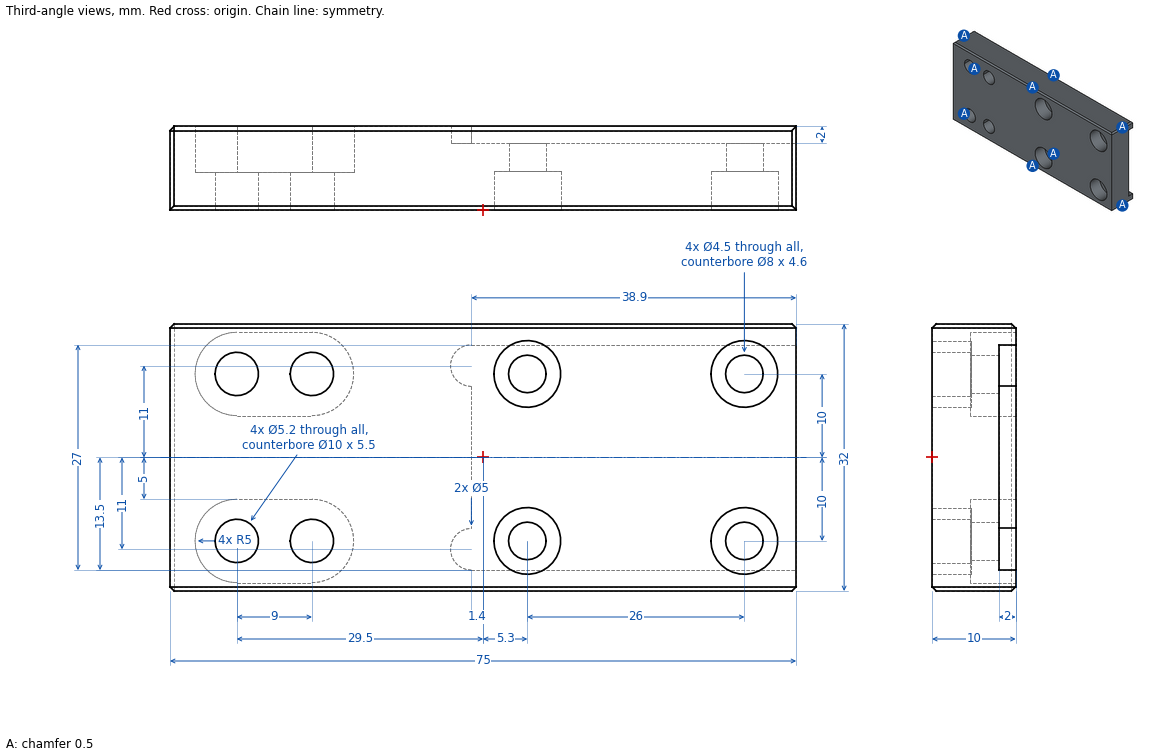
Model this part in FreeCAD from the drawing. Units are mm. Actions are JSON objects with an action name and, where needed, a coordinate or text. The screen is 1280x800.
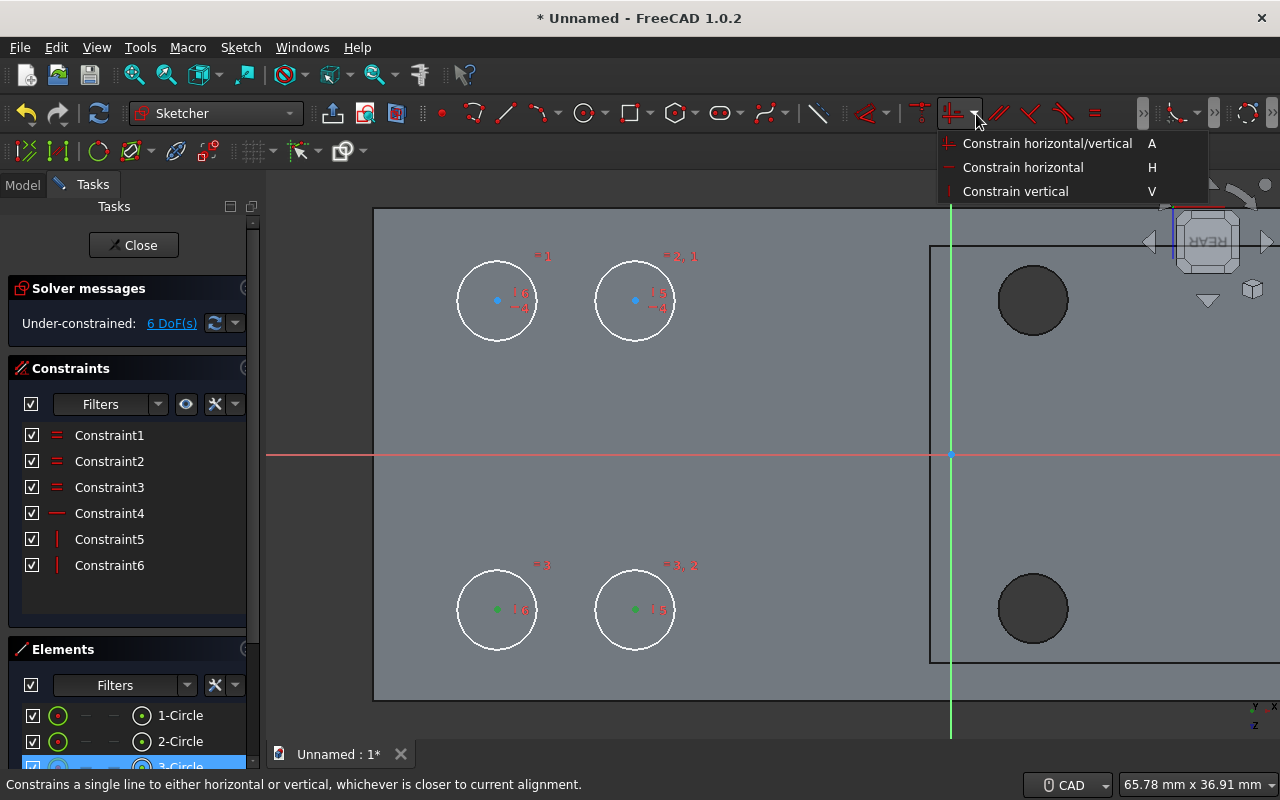
{"action": "left_click", "coordinate": [1073, 167]}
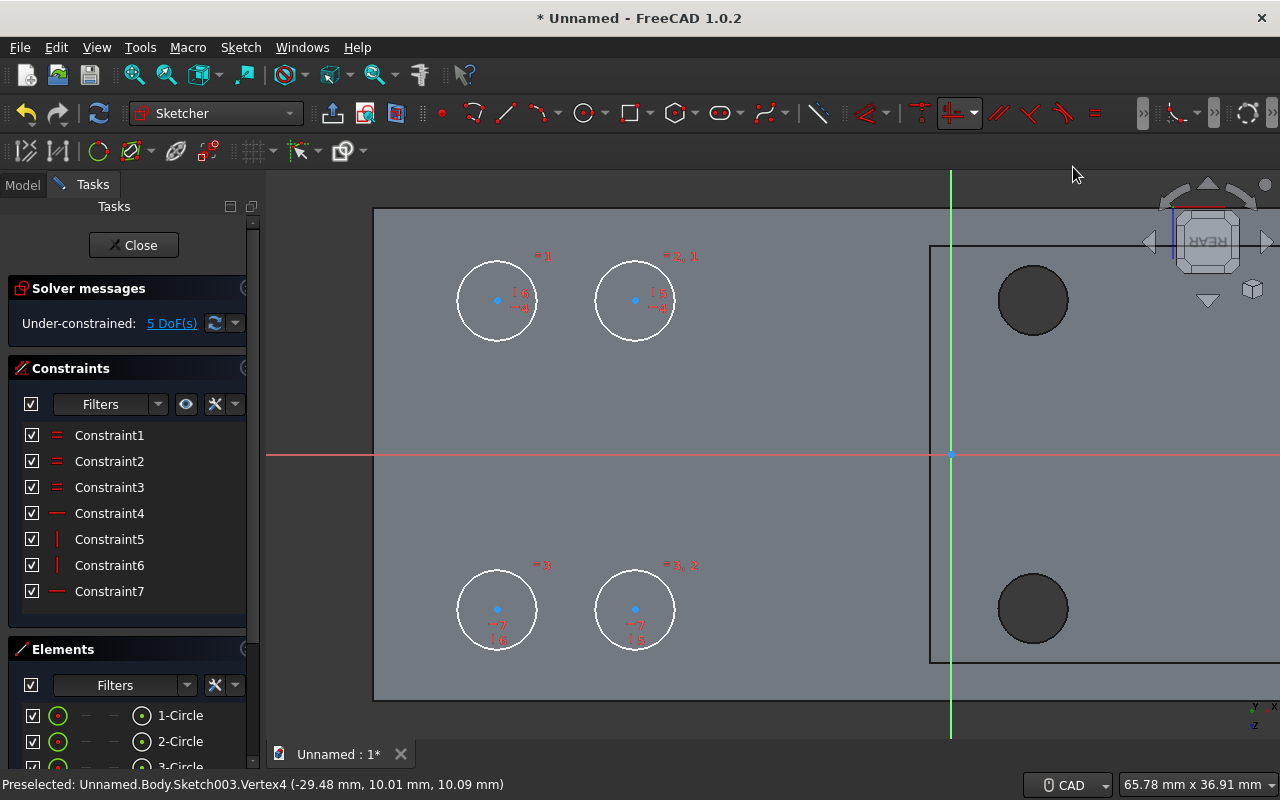
{"action": "left_click", "coordinate": [866, 114]}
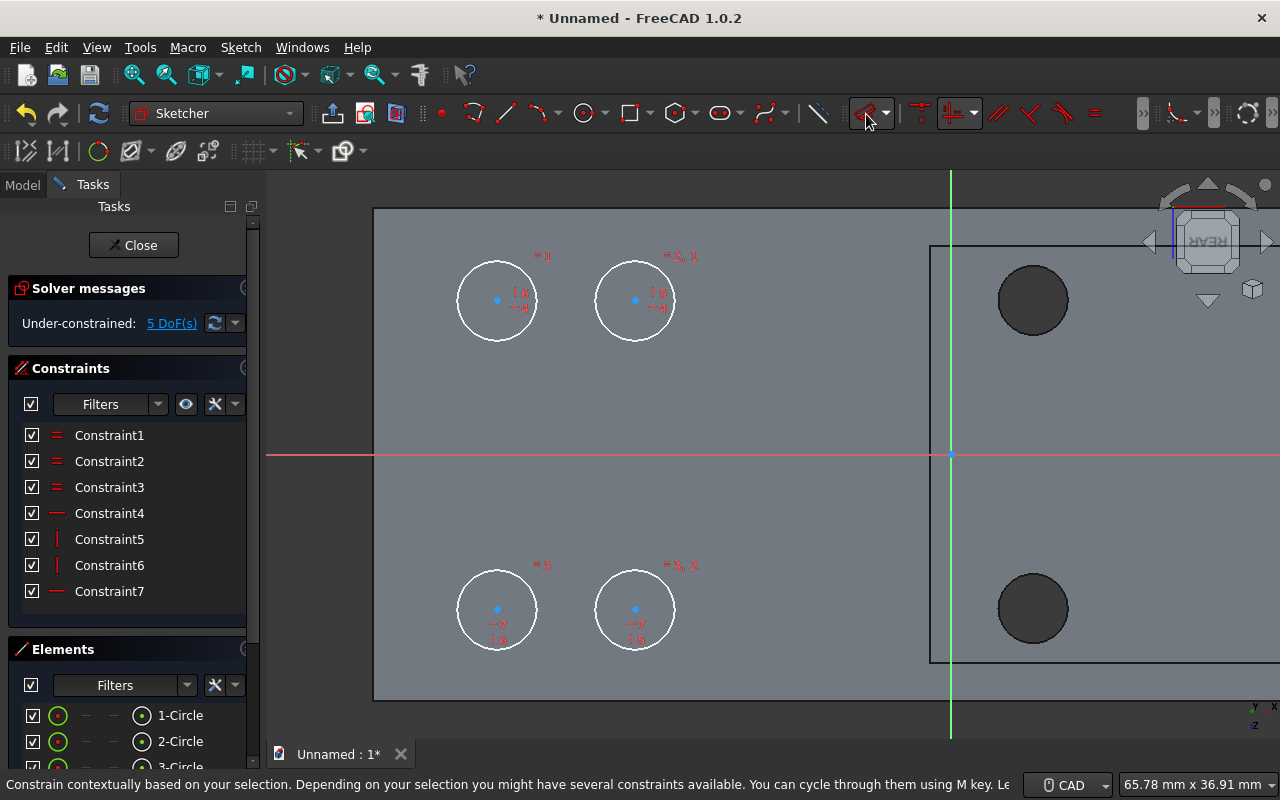
{"action": "left_click", "coordinate": [525, 273]}
{"action": "left_click", "coordinate": [548, 250]}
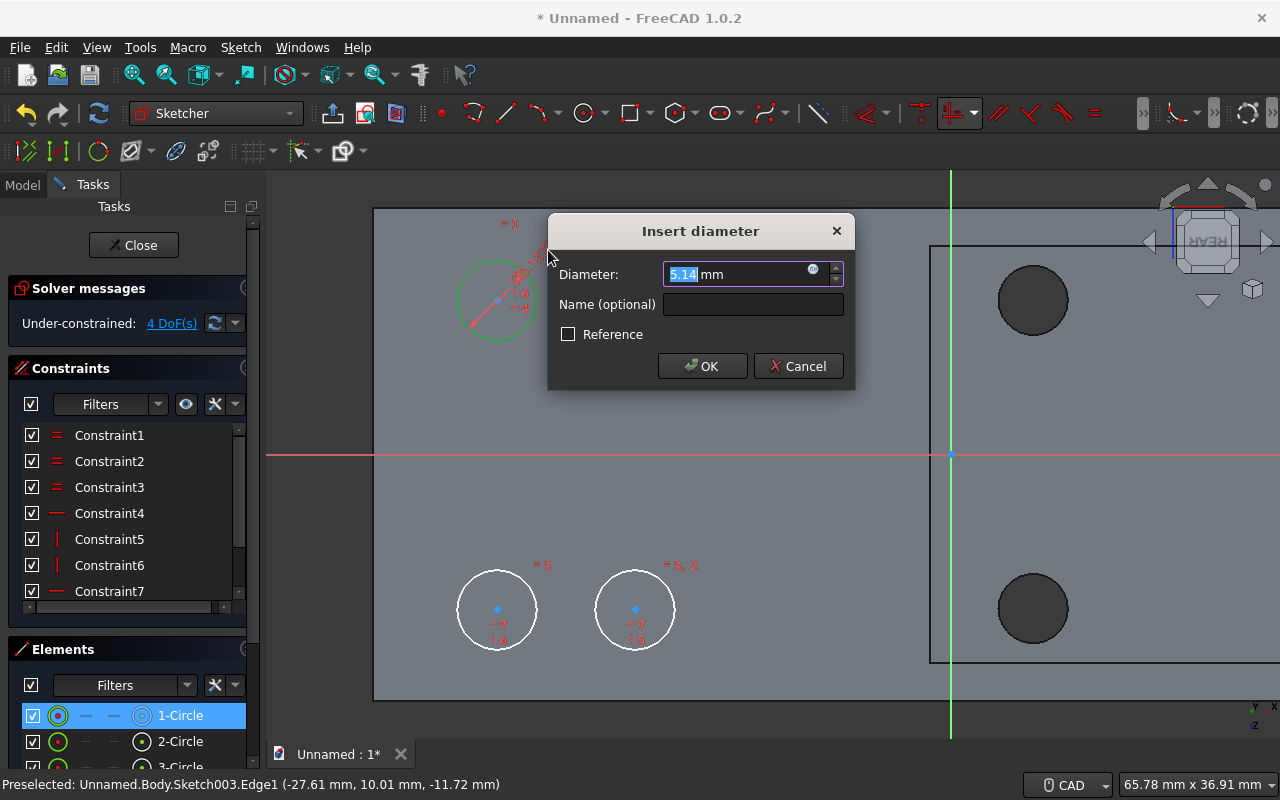
{"action": "type", "text": "5.2"}
{"action": "key", "text": "Return"}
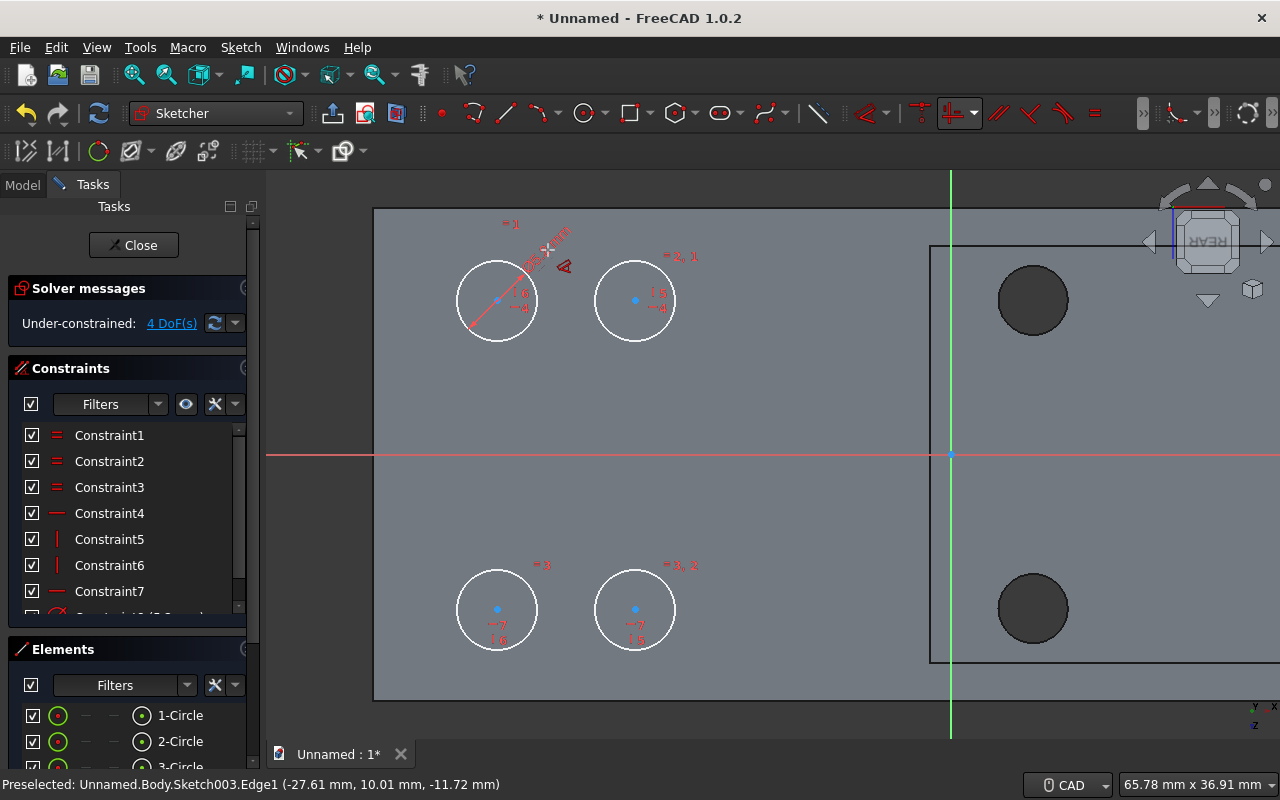
{"action": "left_click", "coordinate": [497, 301]}
{"action": "left_click", "coordinate": [985, 378]}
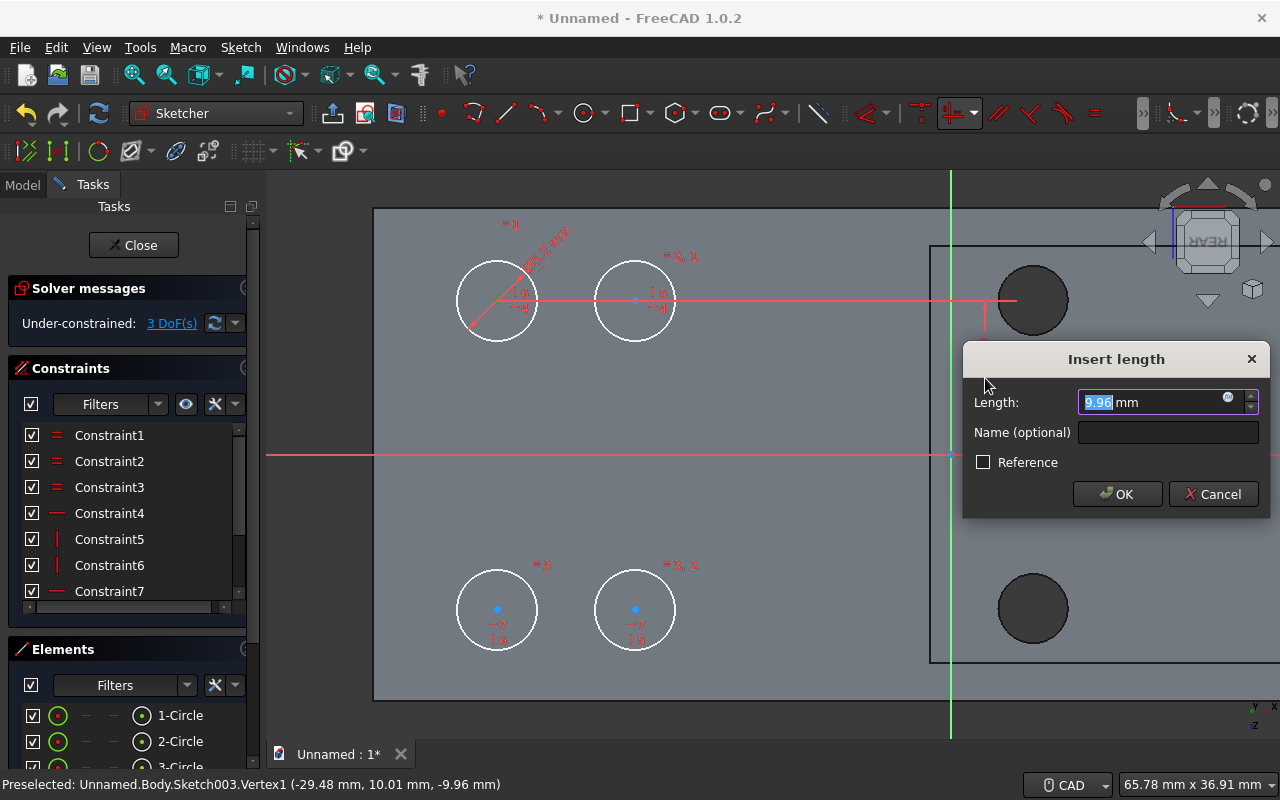
{"action": "type", "text": "10"}
{"action": "key", "text": "Return"}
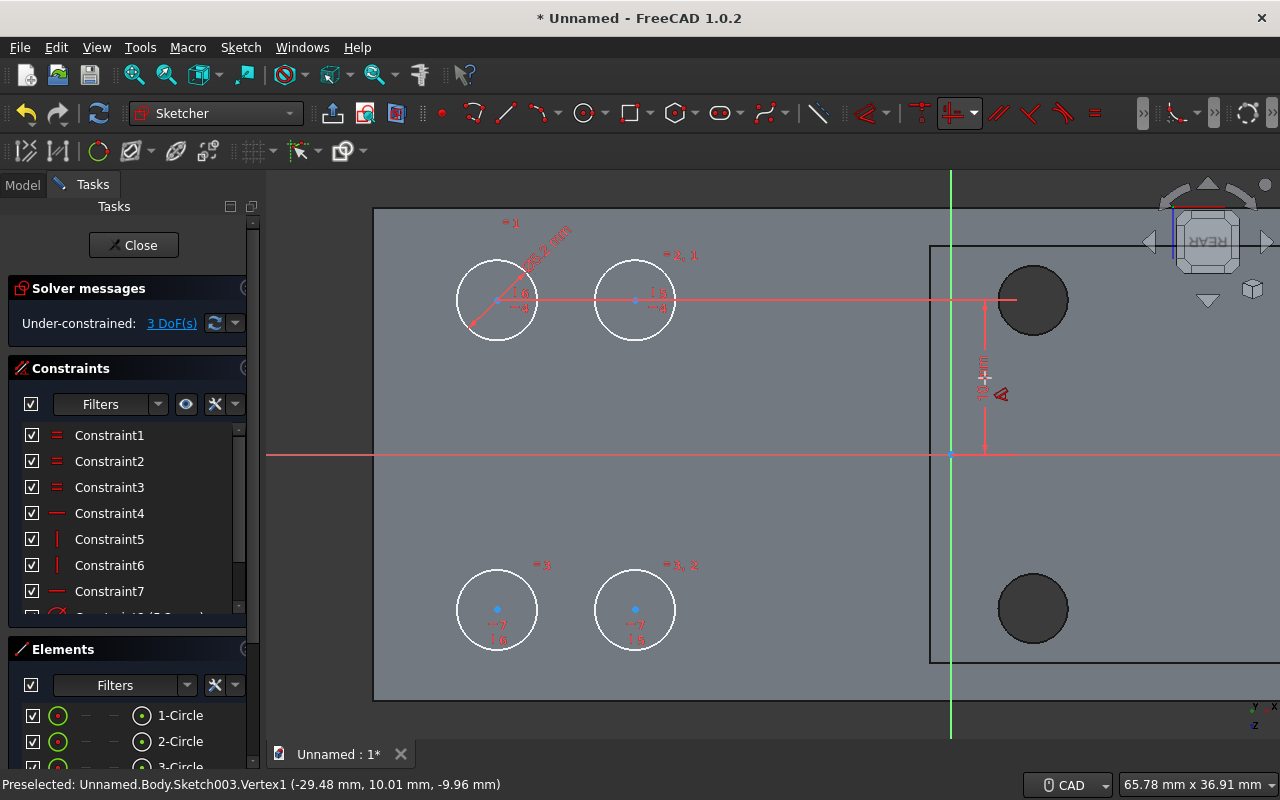
{"action": "left_click", "coordinate": [635, 610]}
{"action": "left_click", "coordinate": [985, 532]}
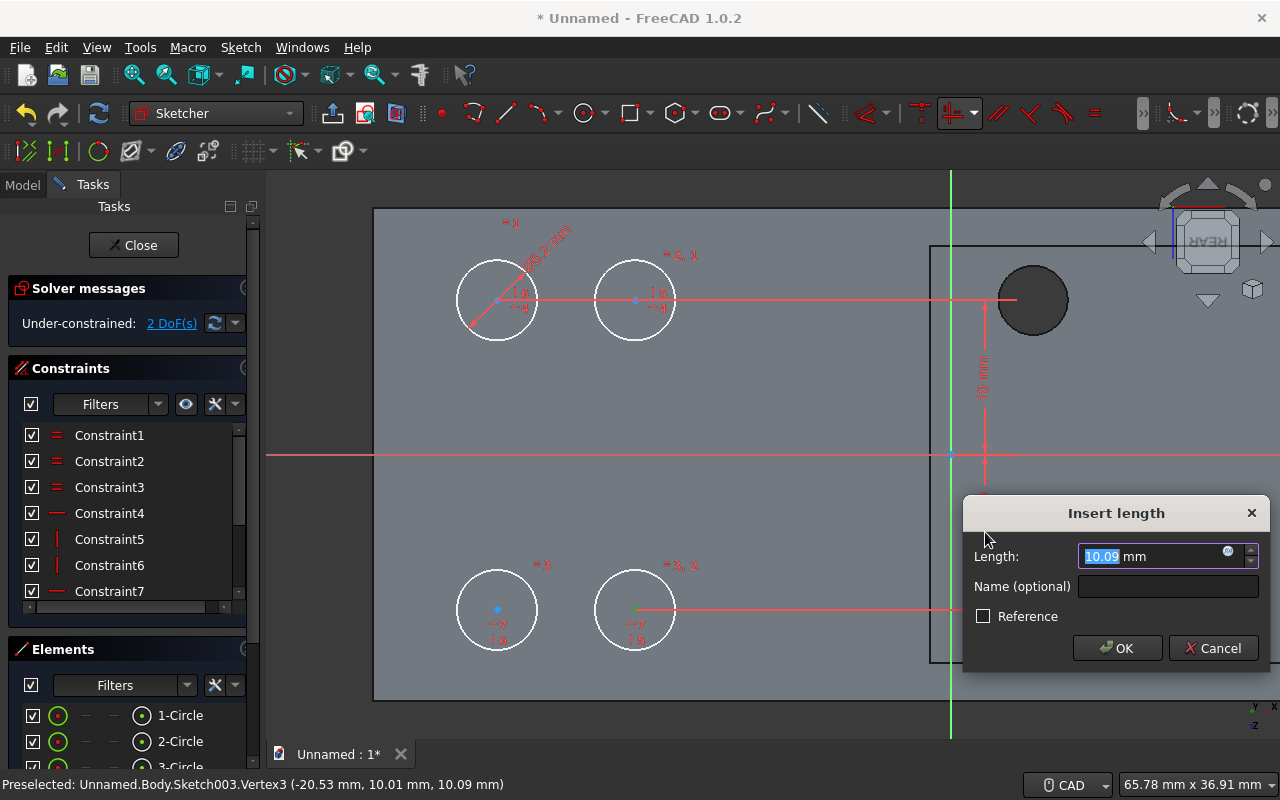
{"action": "type", "text": "10"}
{"action": "key", "text": "Return"}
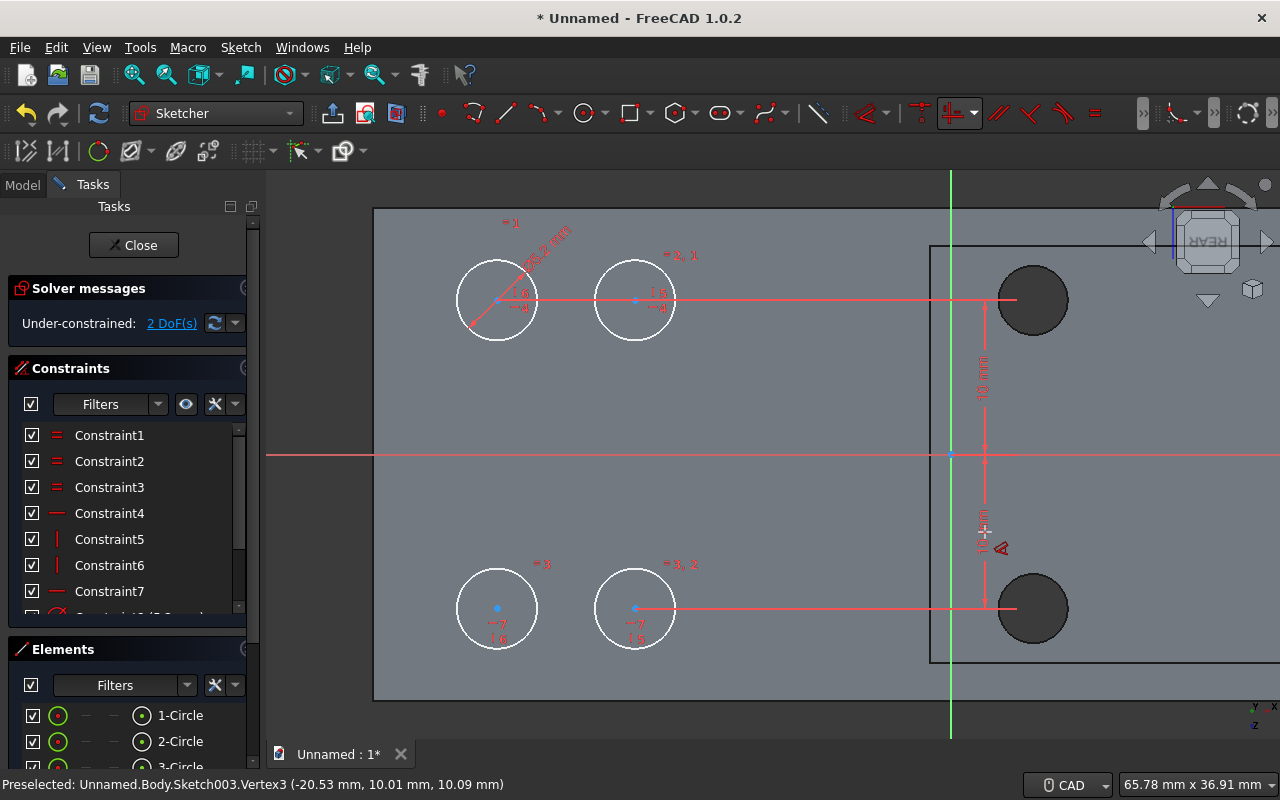
{"action": "left_click", "coordinate": [497, 300]}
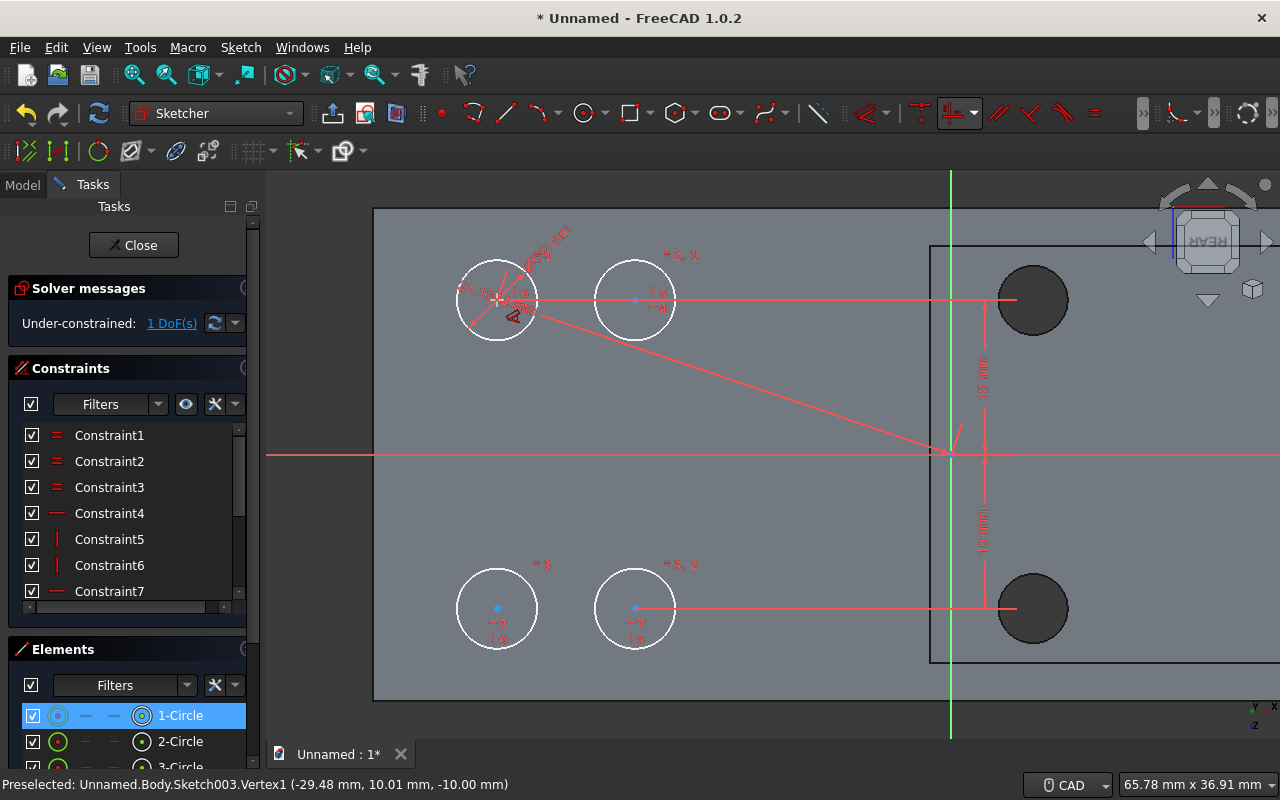
{"action": "left_click", "coordinate": [635, 300]}
{"action": "left_click", "coordinate": [566, 334]}